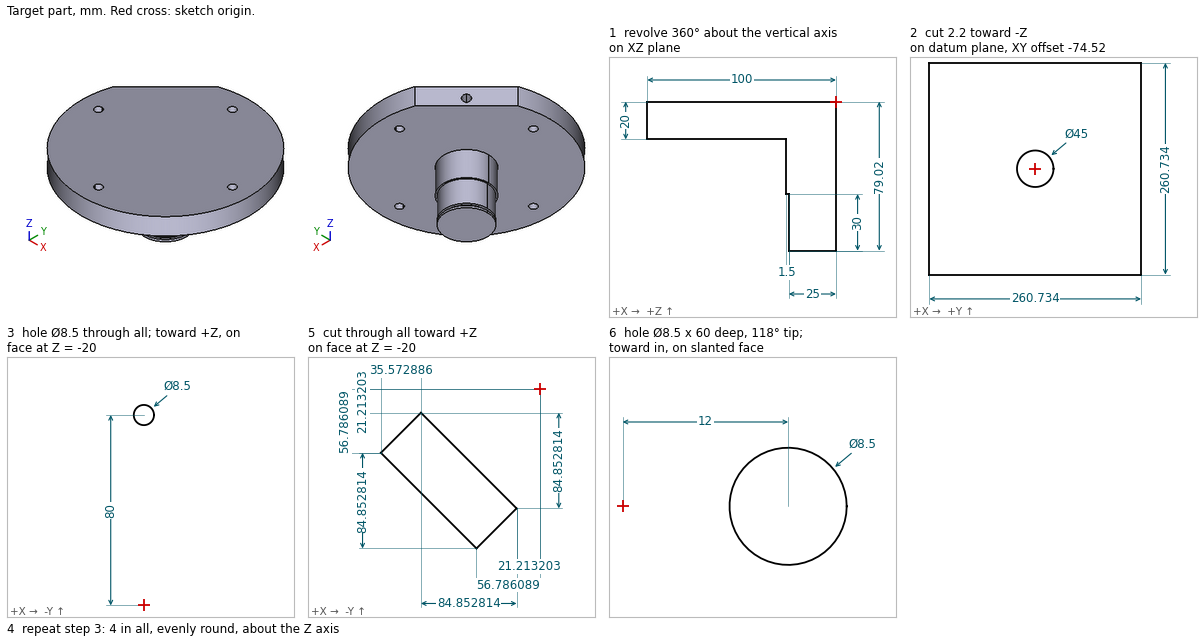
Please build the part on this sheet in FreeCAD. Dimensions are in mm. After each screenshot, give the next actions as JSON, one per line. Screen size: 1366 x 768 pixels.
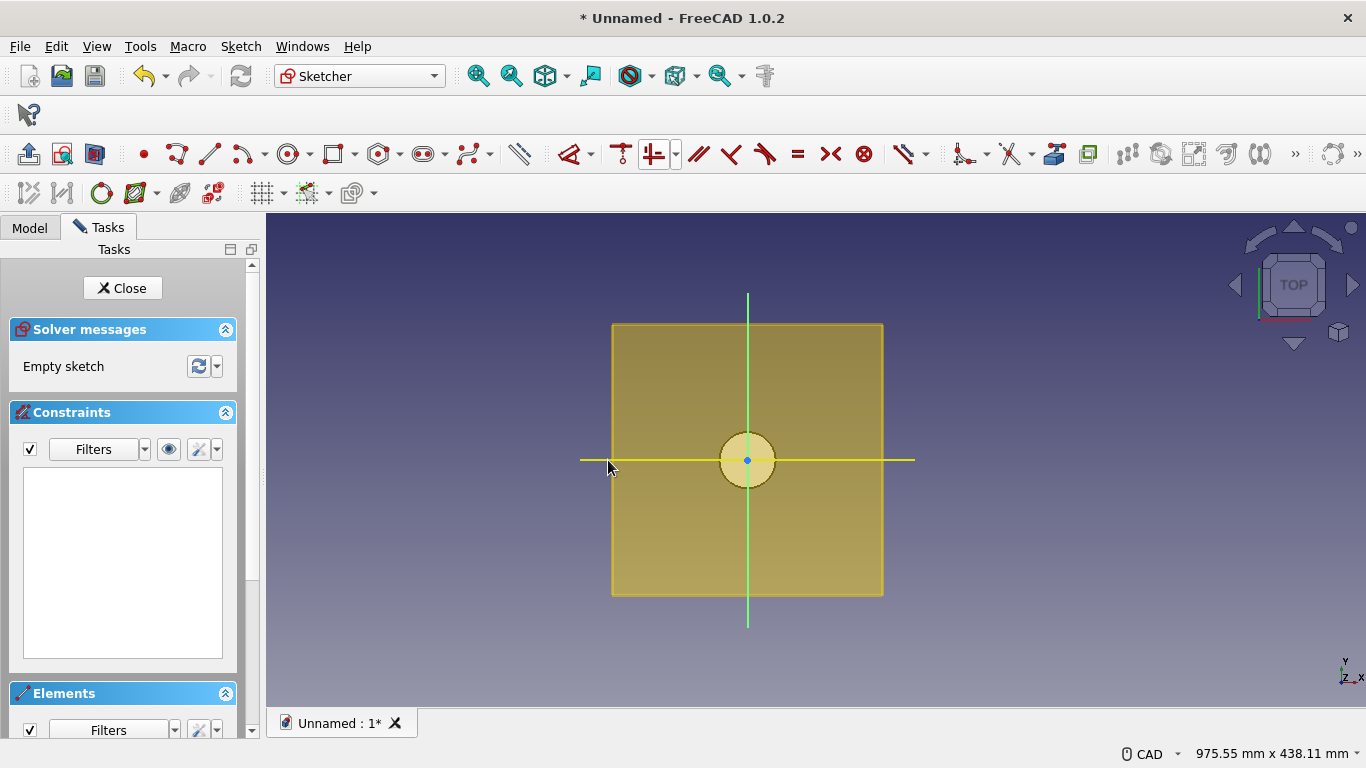
{"action": "left_click", "coordinate": [354, 154]}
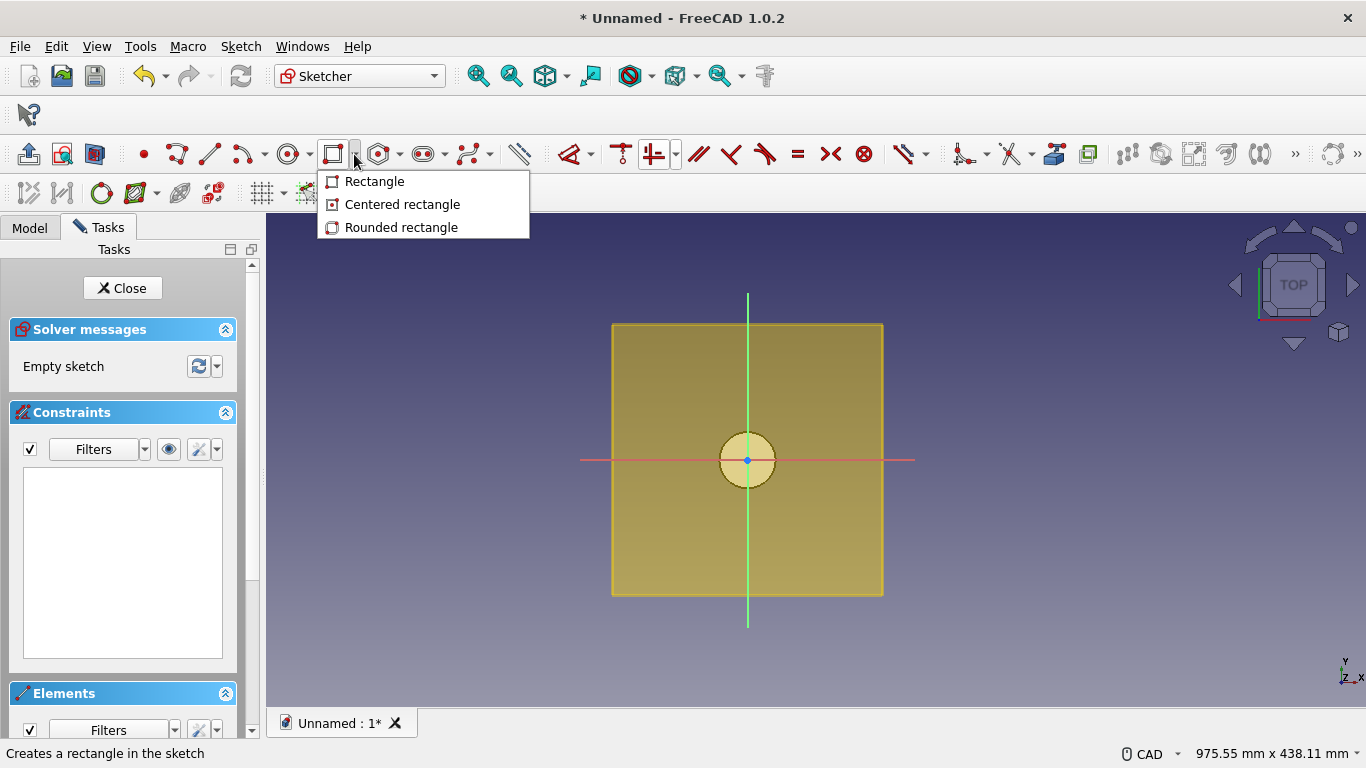
{"action": "left_click", "coordinate": [424, 204]}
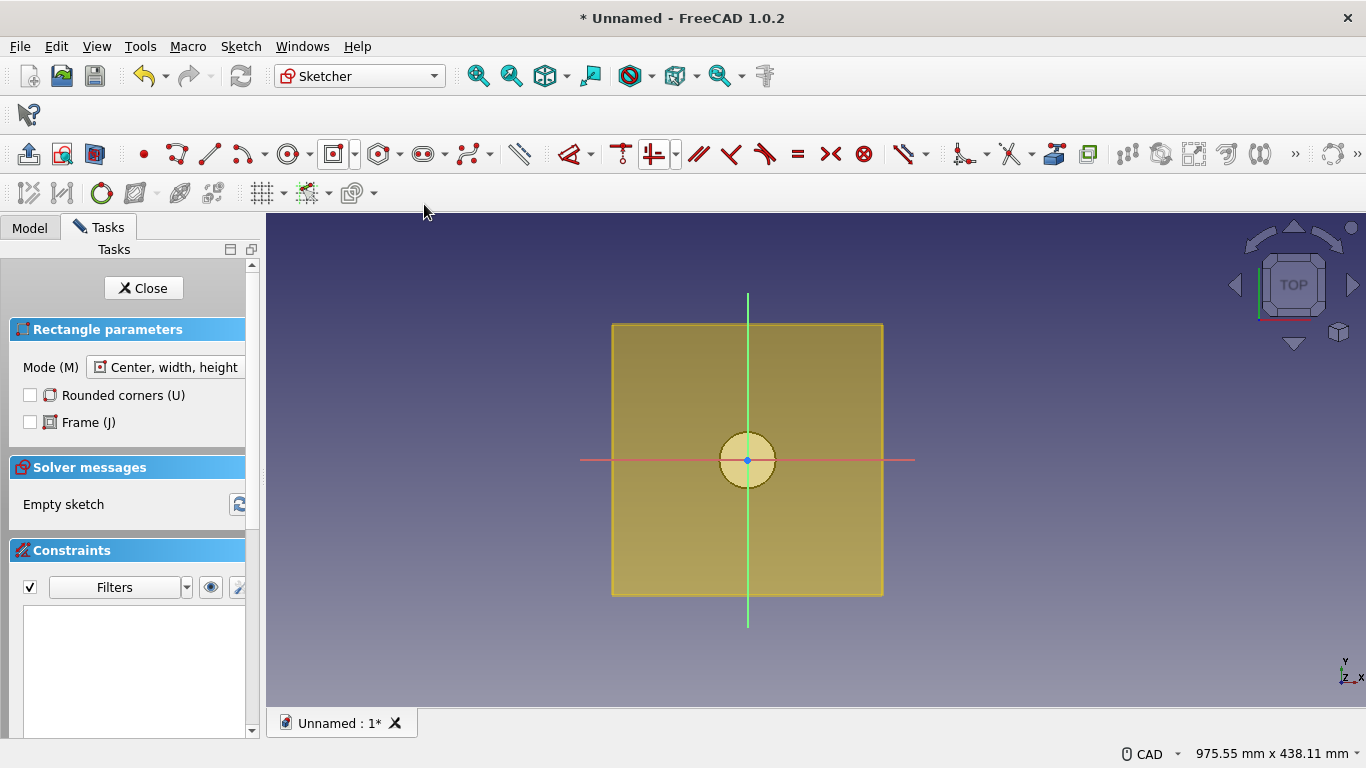
{"action": "left_click", "coordinate": [748, 460]}
{"action": "mouse_move", "coordinate": [895, 313]}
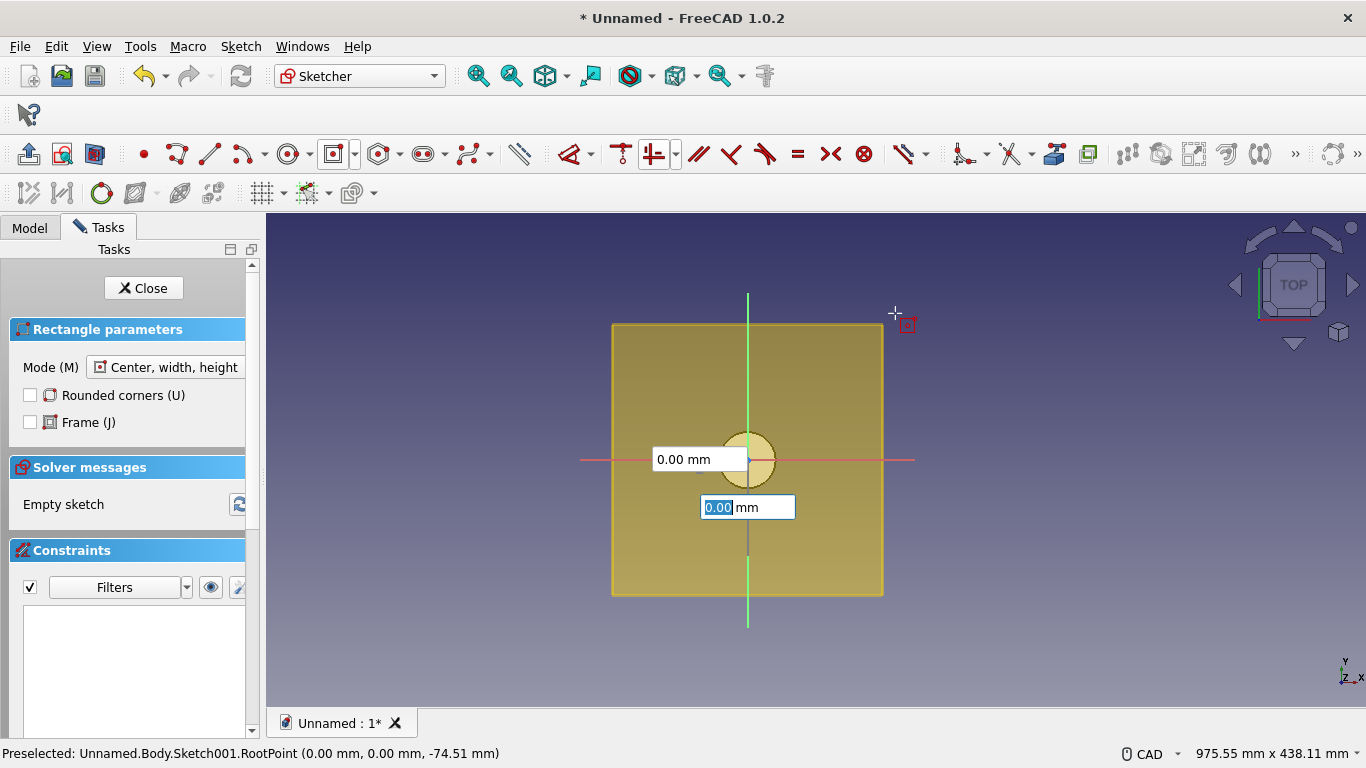
{"action": "type", "text": "260.734"}
{"action": "key", "text": "Tab"}
{"action": "type", "text": "260.734"}
{"action": "key", "text": "Return"}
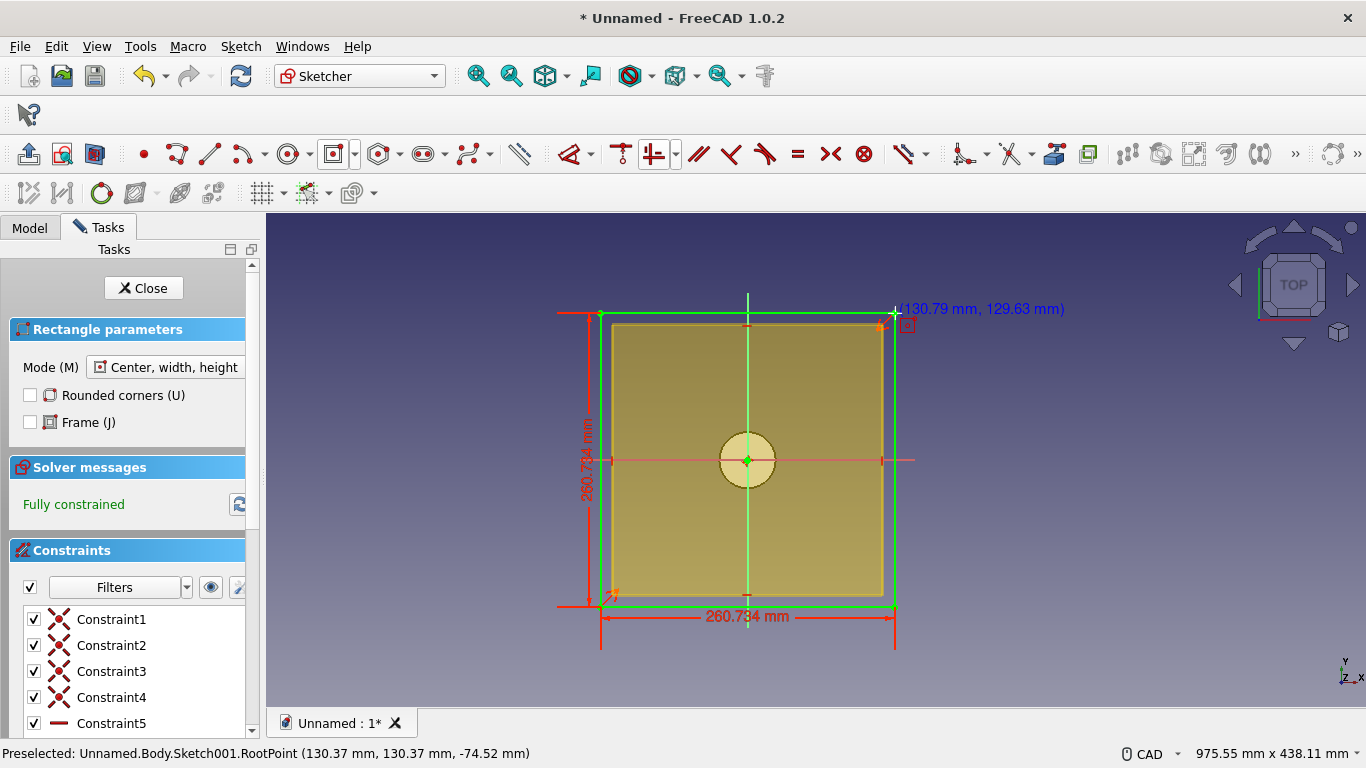
{"action": "left_click", "coordinate": [288, 154]}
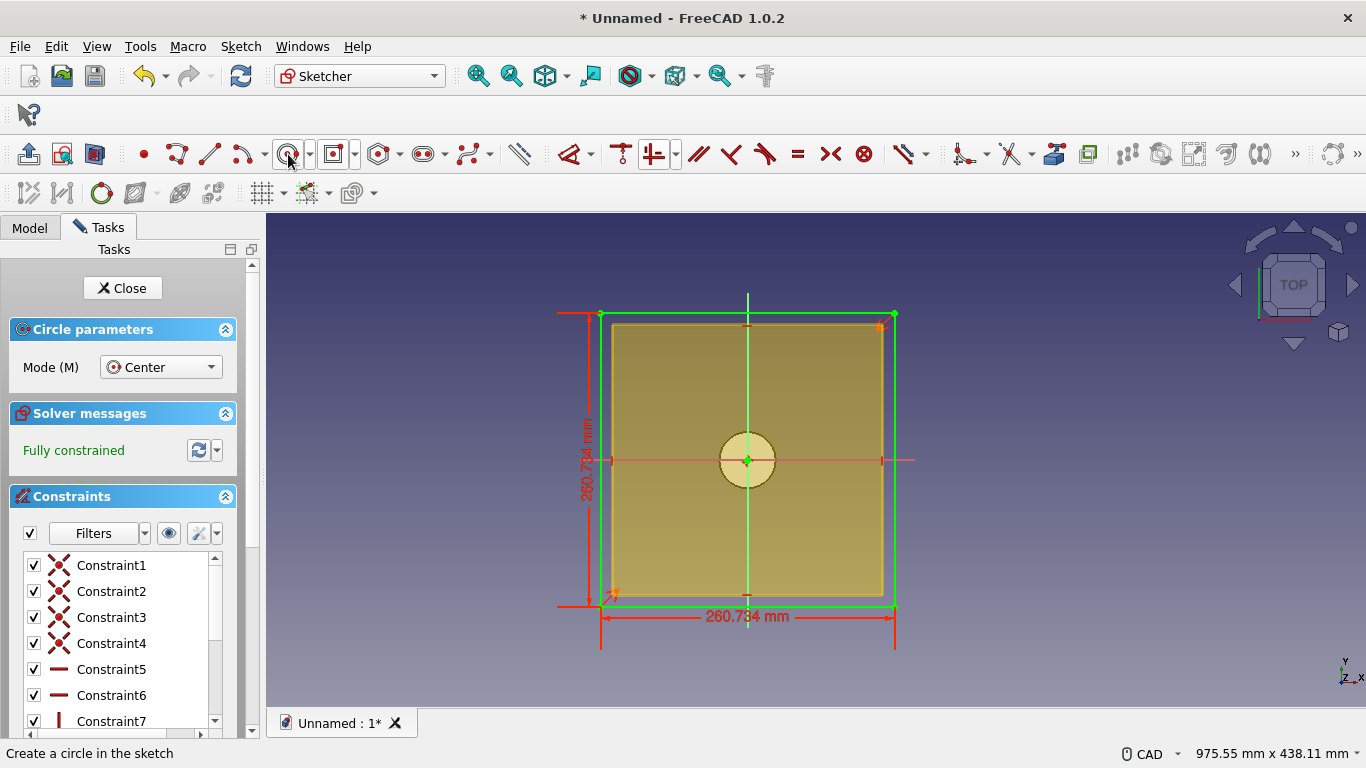
{"action": "left_click", "coordinate": [748, 460]}
{"action": "mouse_move", "coordinate": [765, 442]}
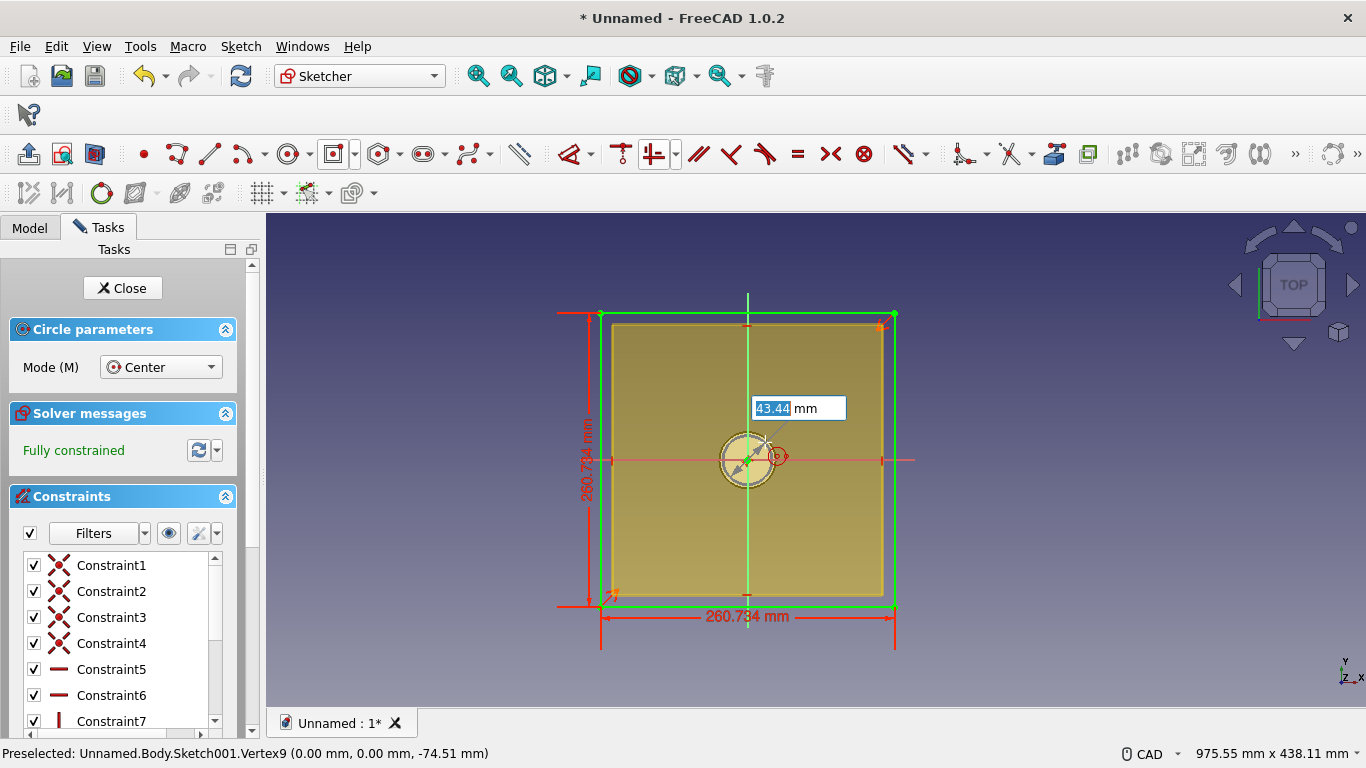
{"action": "type", "text": "45"}
{"action": "key", "text": "Return"}
{"action": "key", "text": "Escape"}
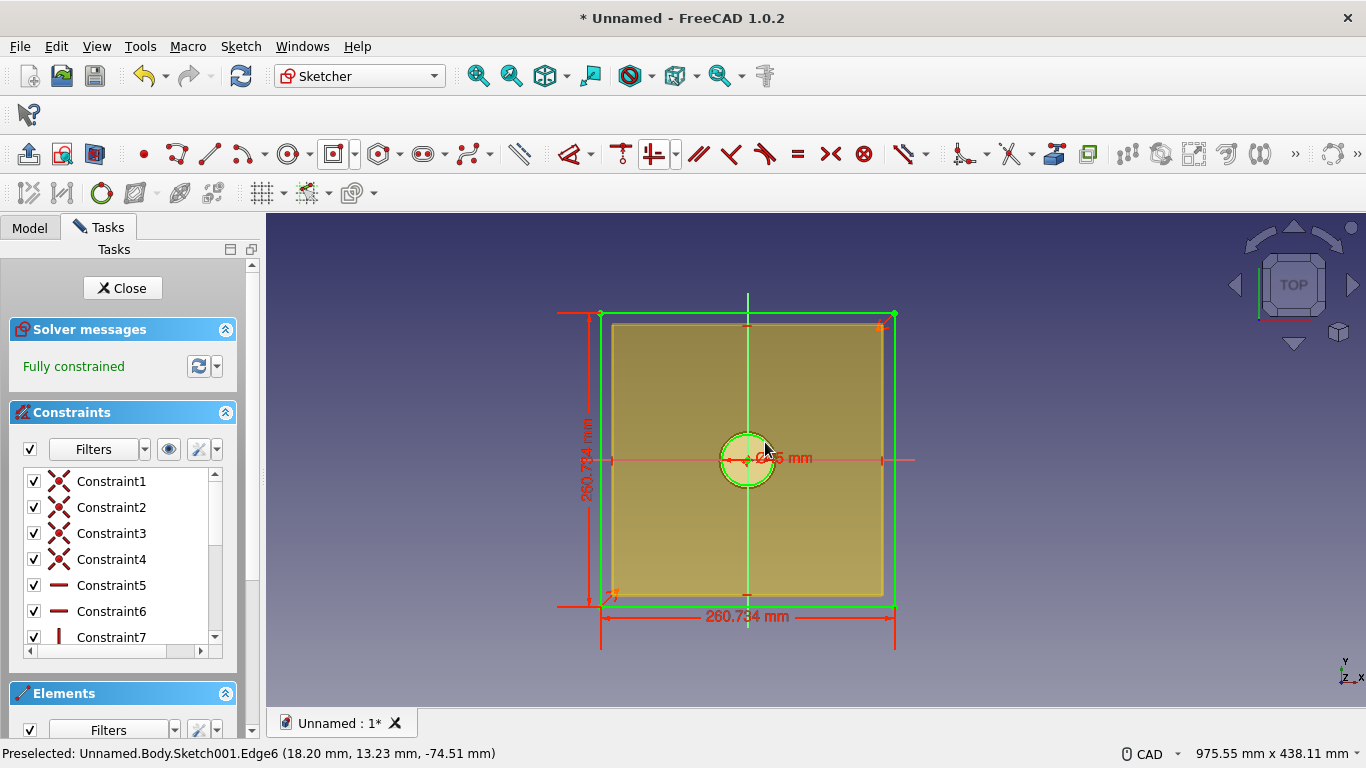
{"action": "left_click", "coordinate": [123, 288]}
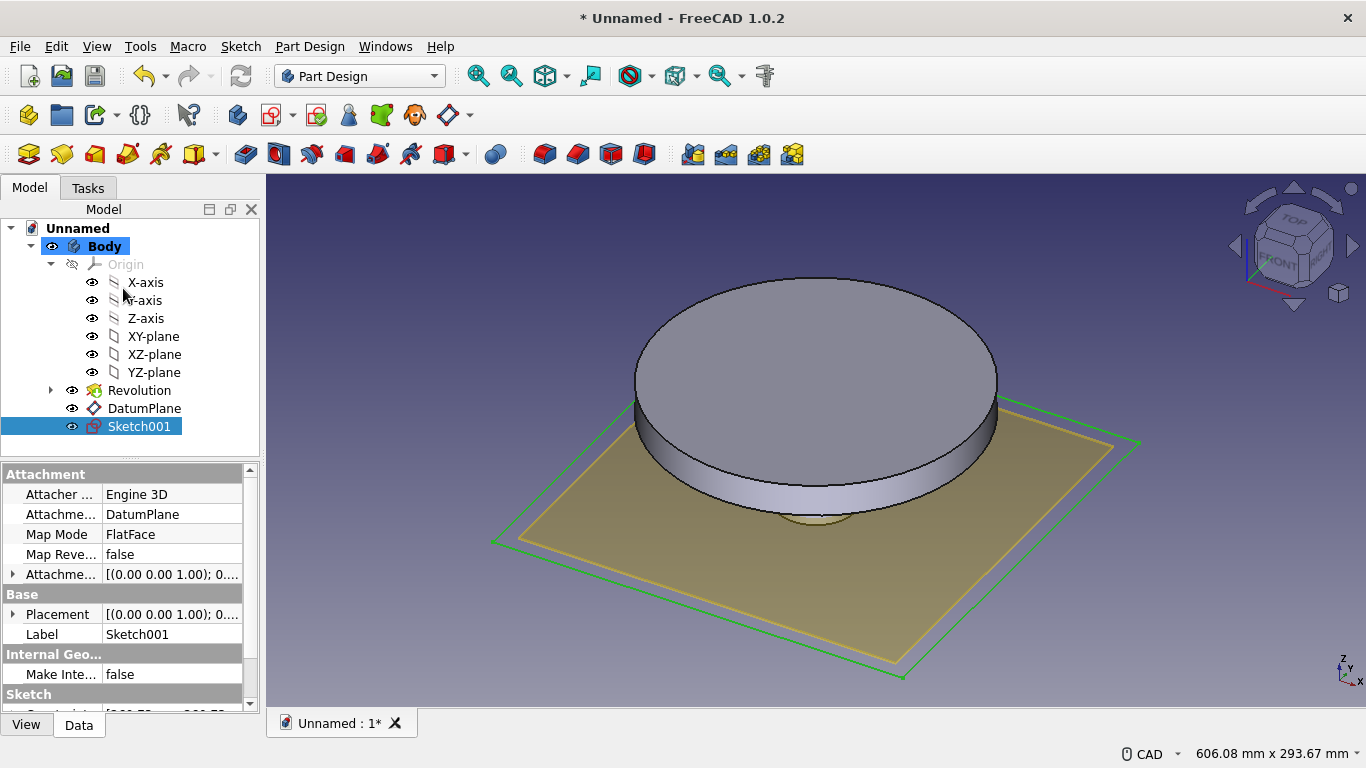
{"action": "left_click", "coordinate": [246, 154]}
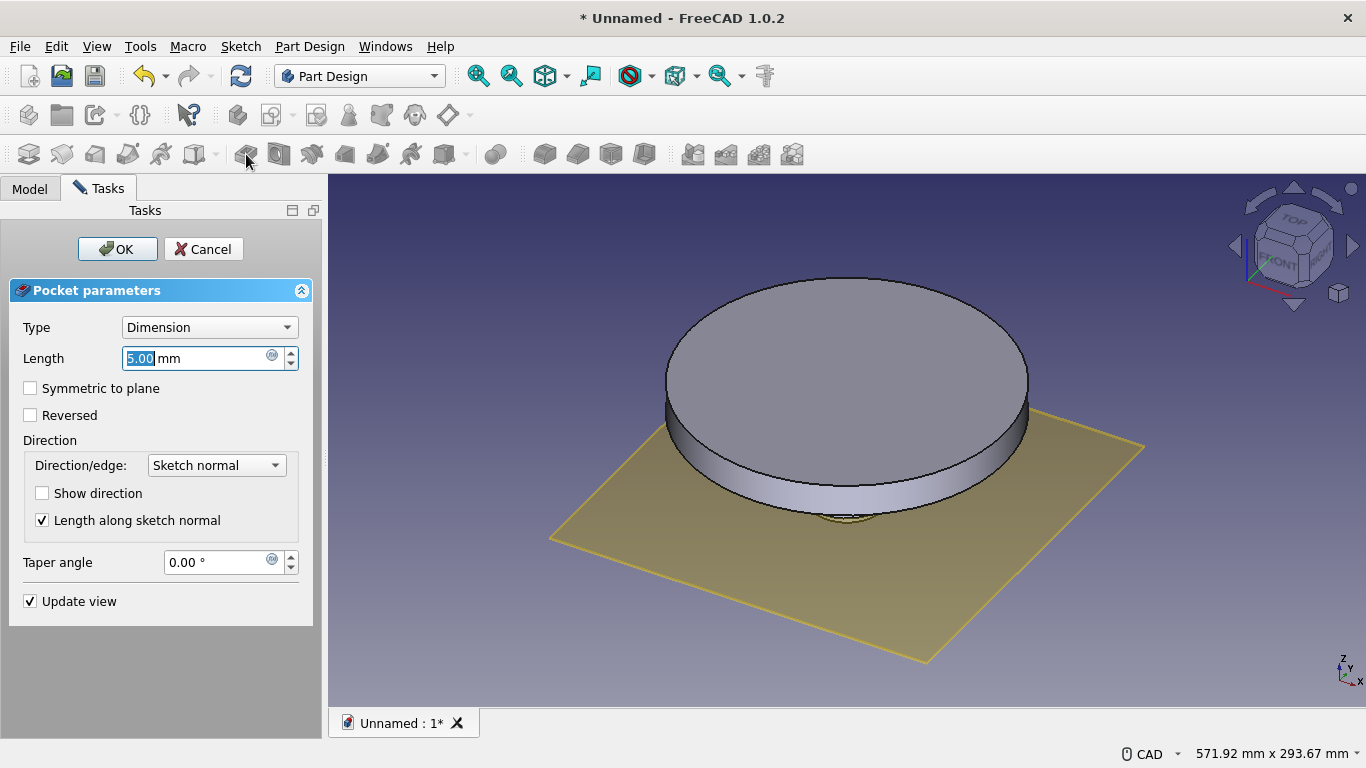
{"action": "type", "text": "2.2"}
{"action": "key", "text": "Tab"}